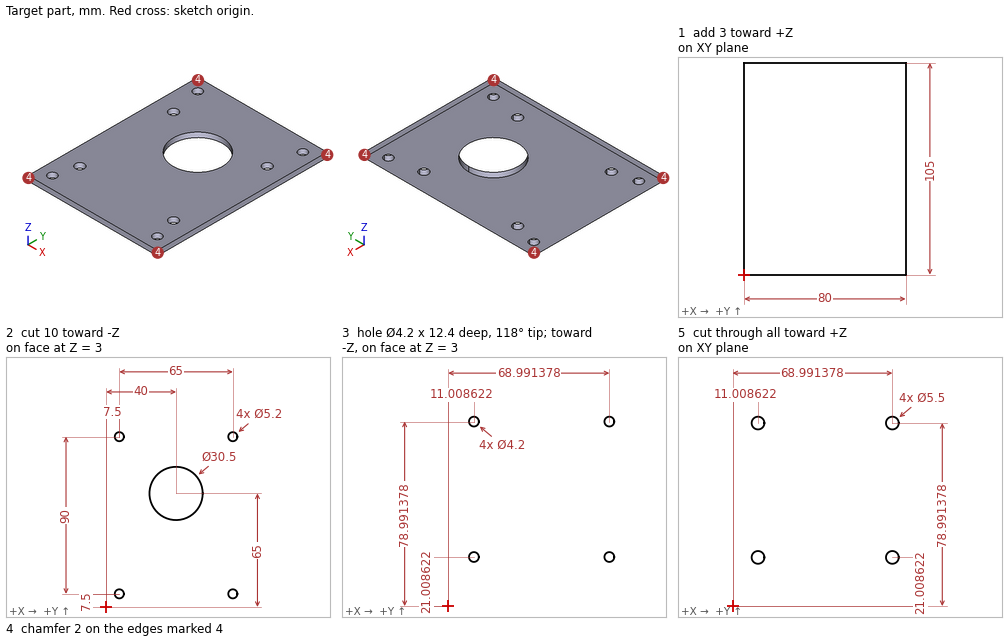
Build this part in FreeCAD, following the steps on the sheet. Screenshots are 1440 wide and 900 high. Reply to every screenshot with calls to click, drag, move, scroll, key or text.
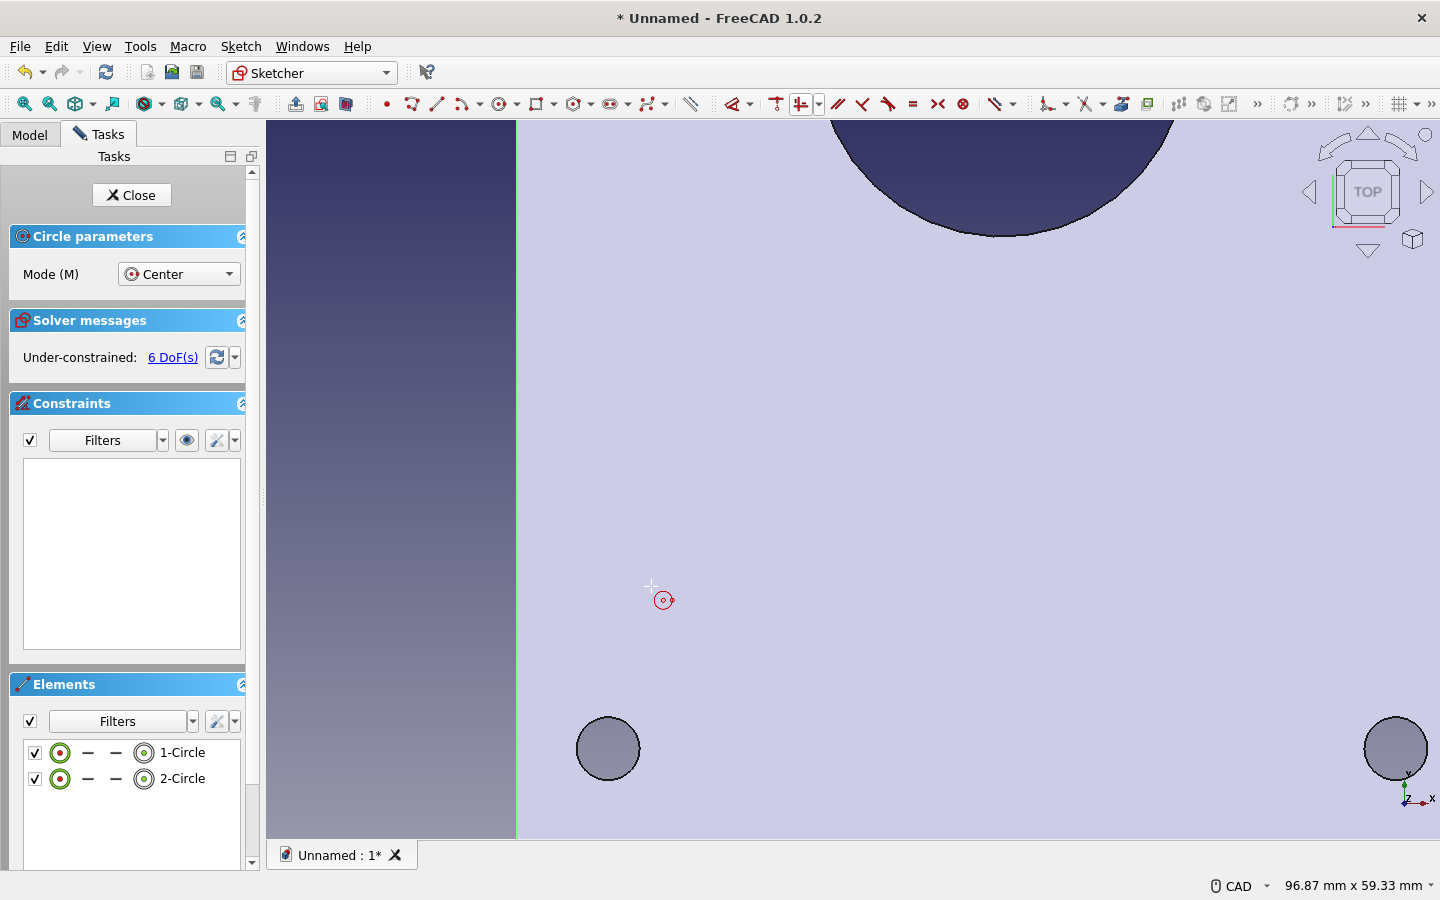
click(651, 585)
click(669, 567)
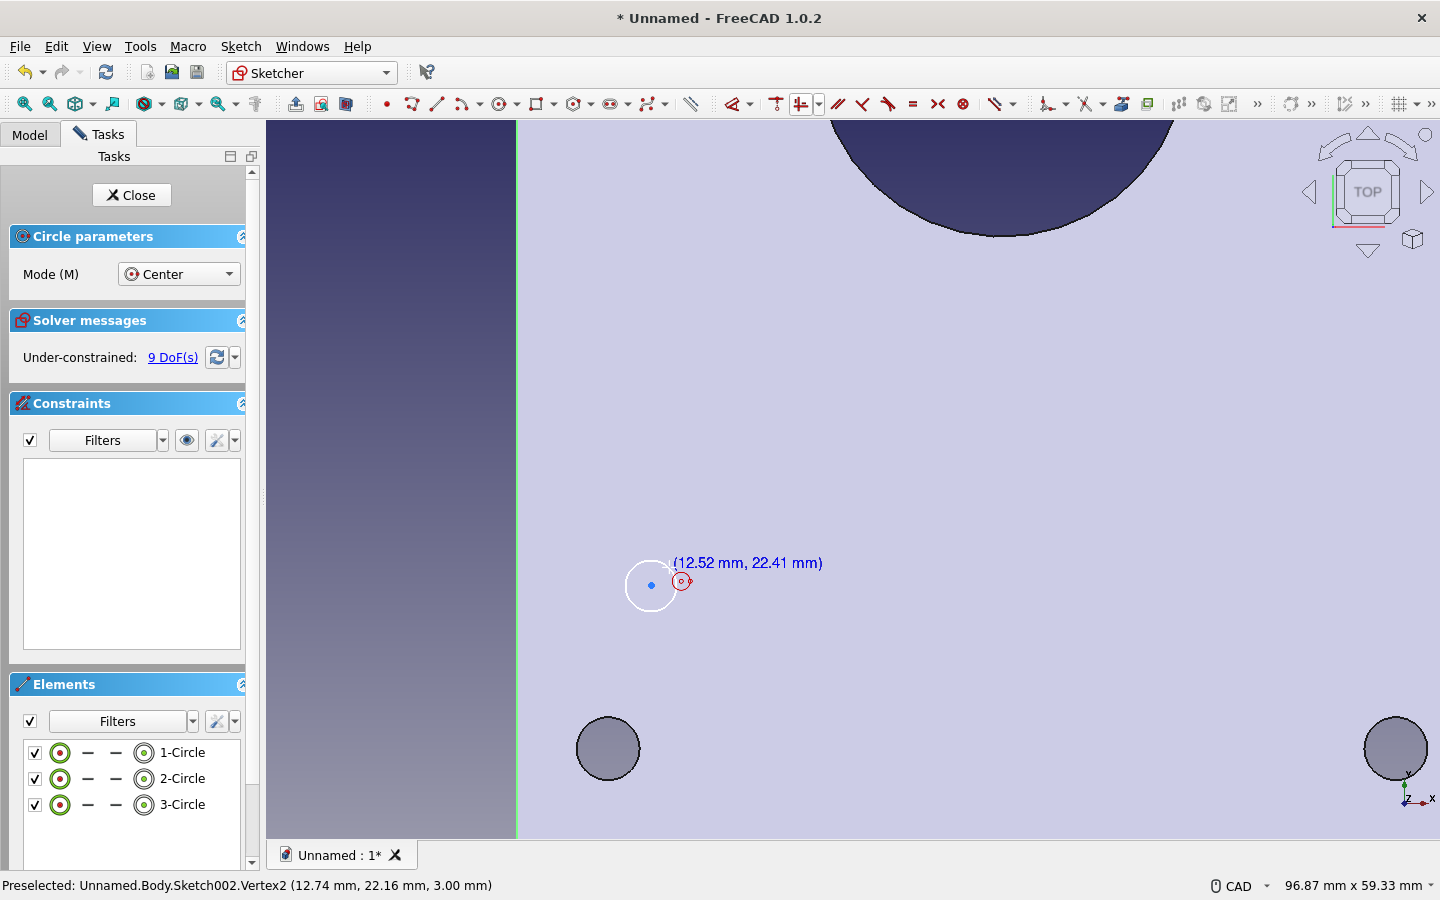
scroll(651, 587, down, 4)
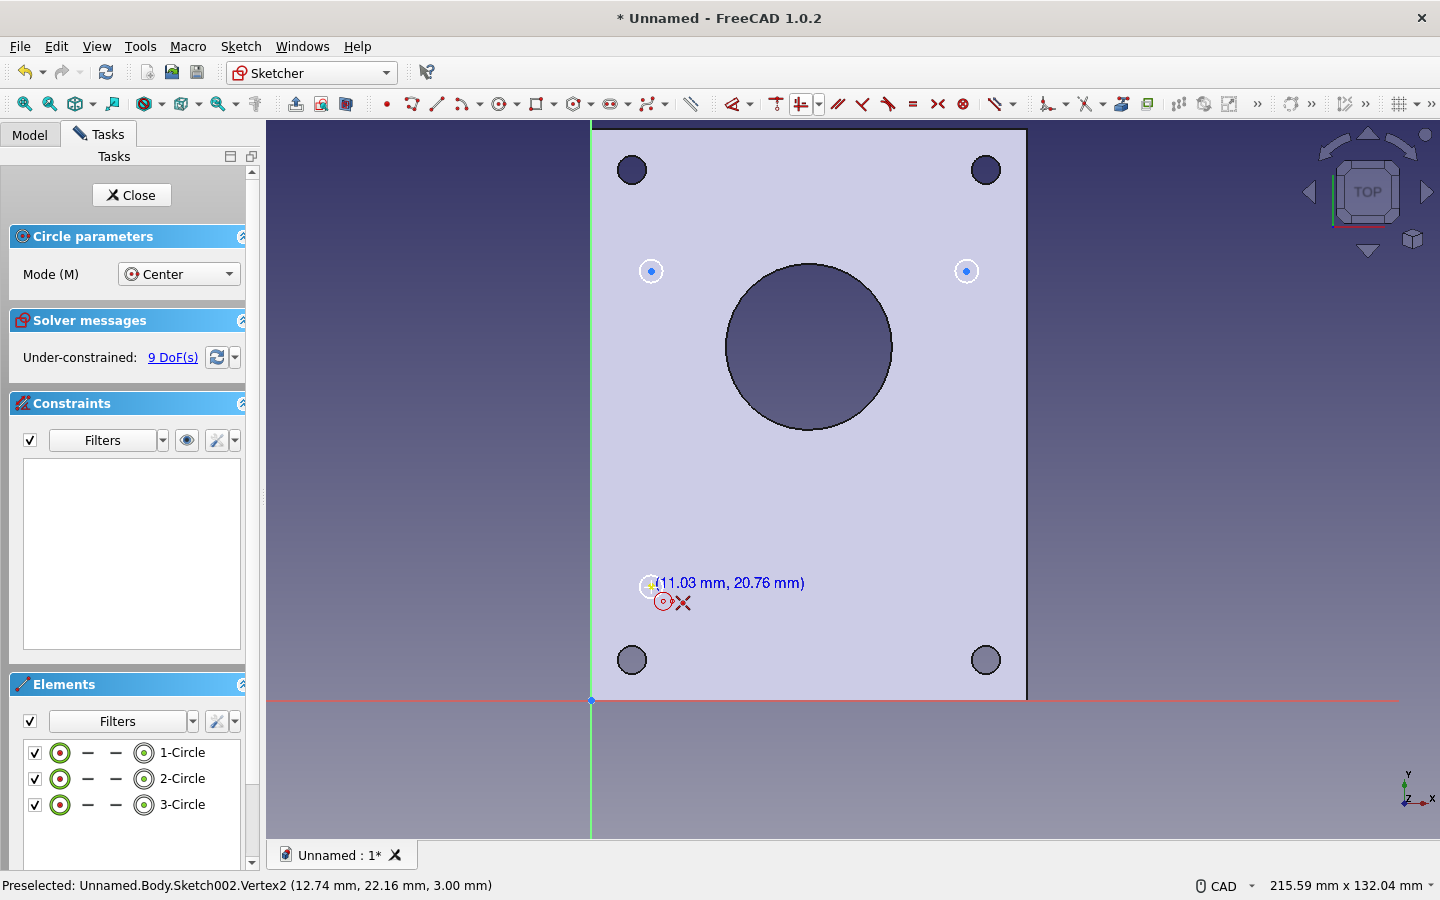
scroll(967, 586, up, 4)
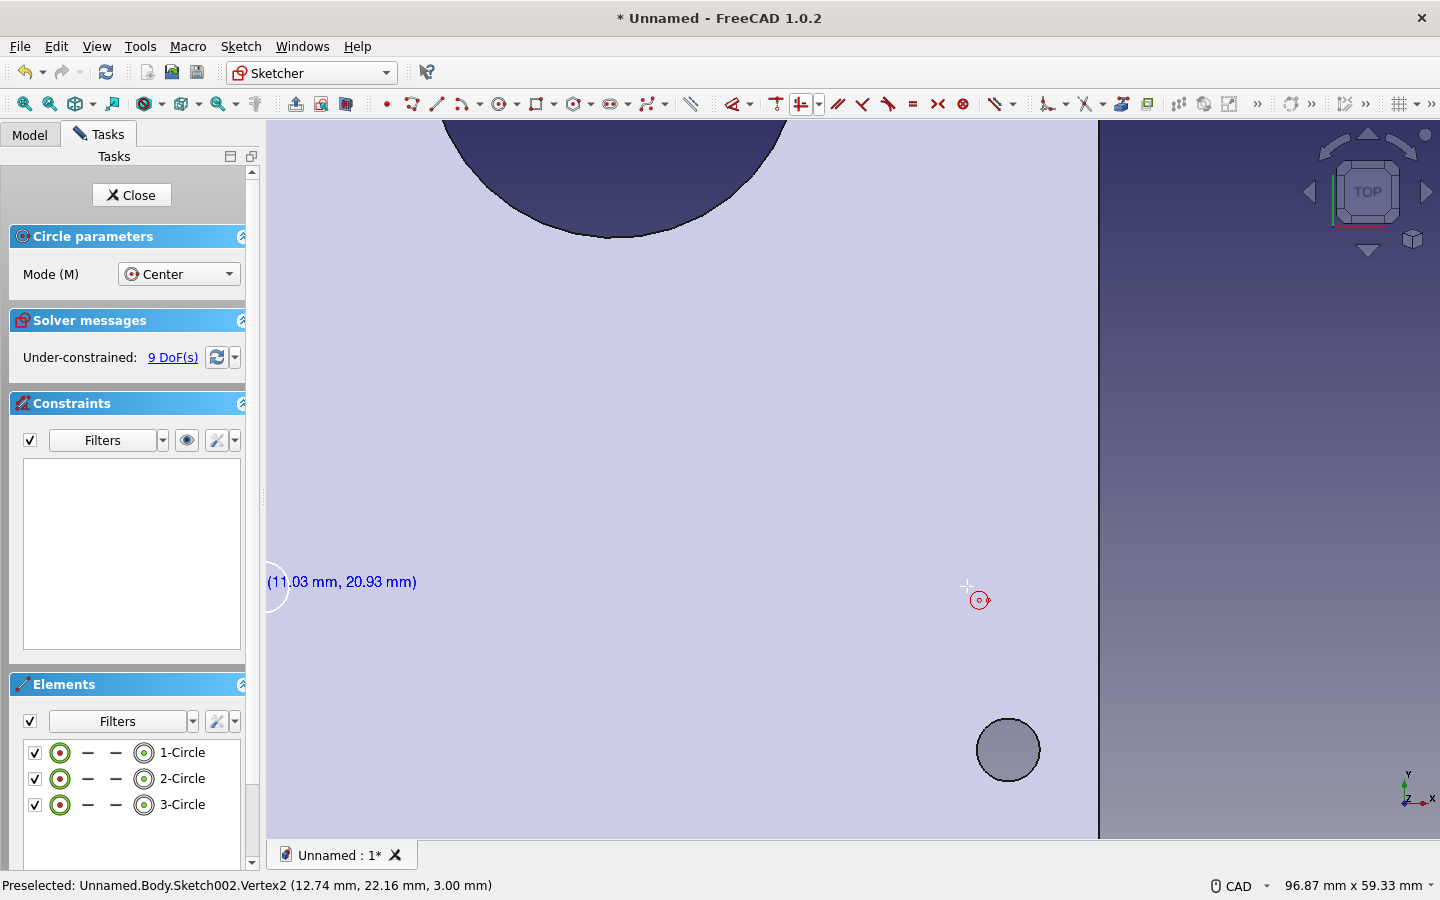
click(966, 586)
click(984, 568)
key(Escape)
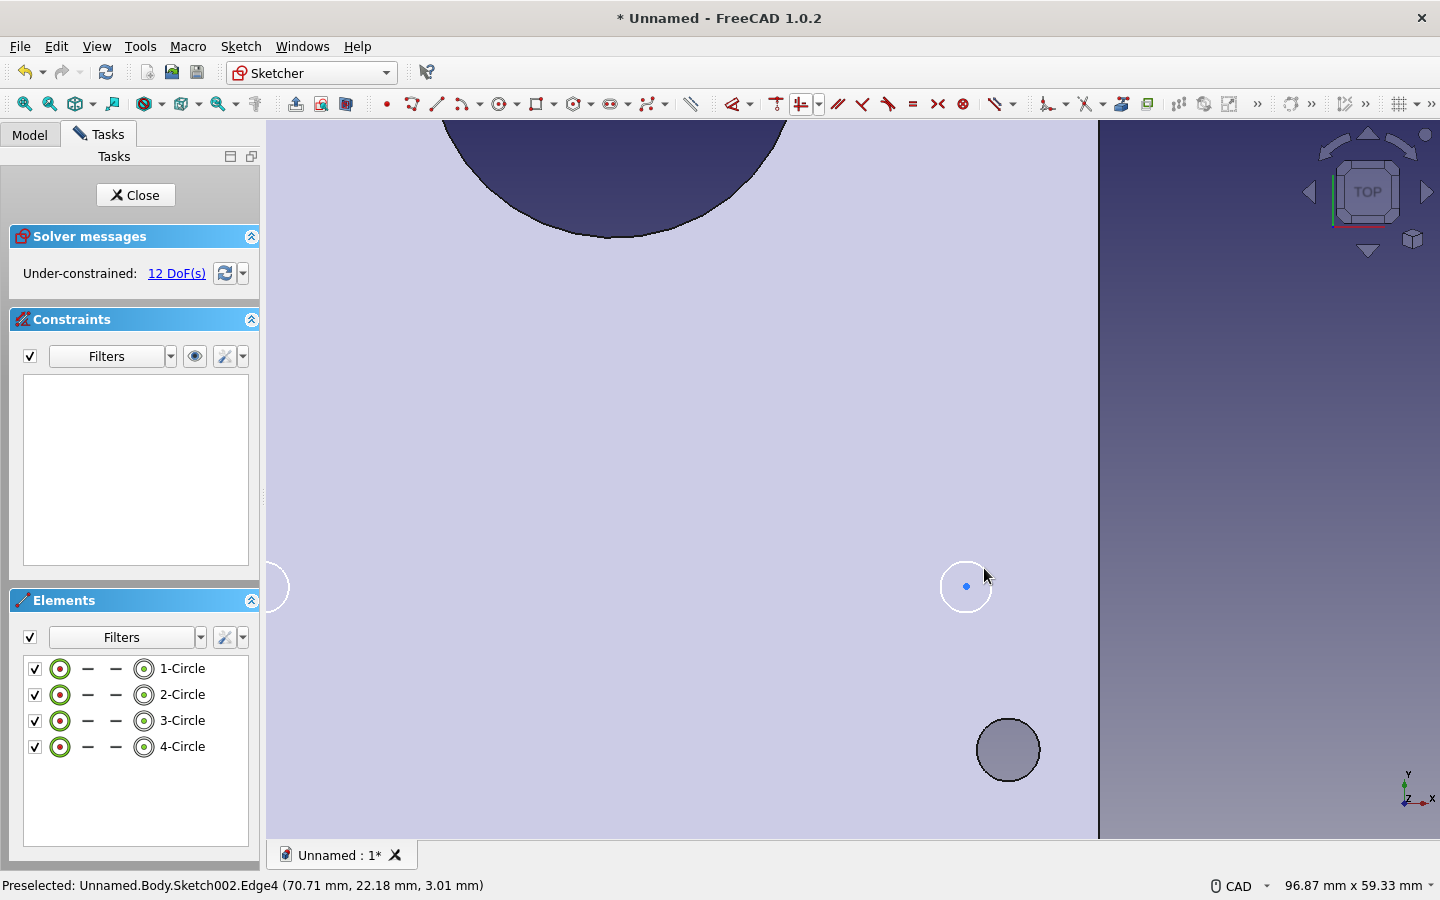
scroll(967, 586, down, 4)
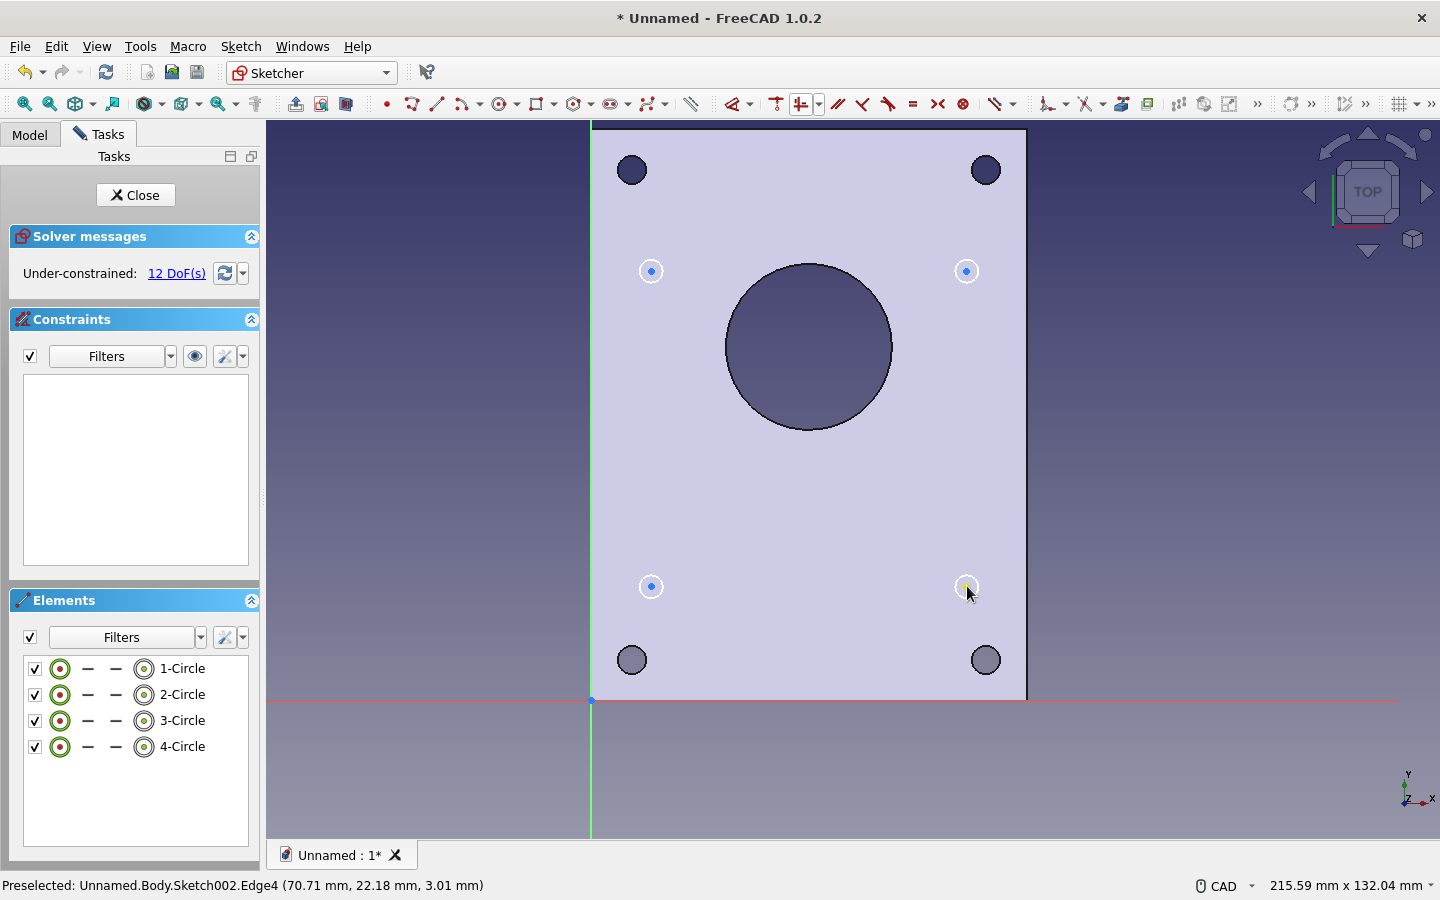
click(659, 263)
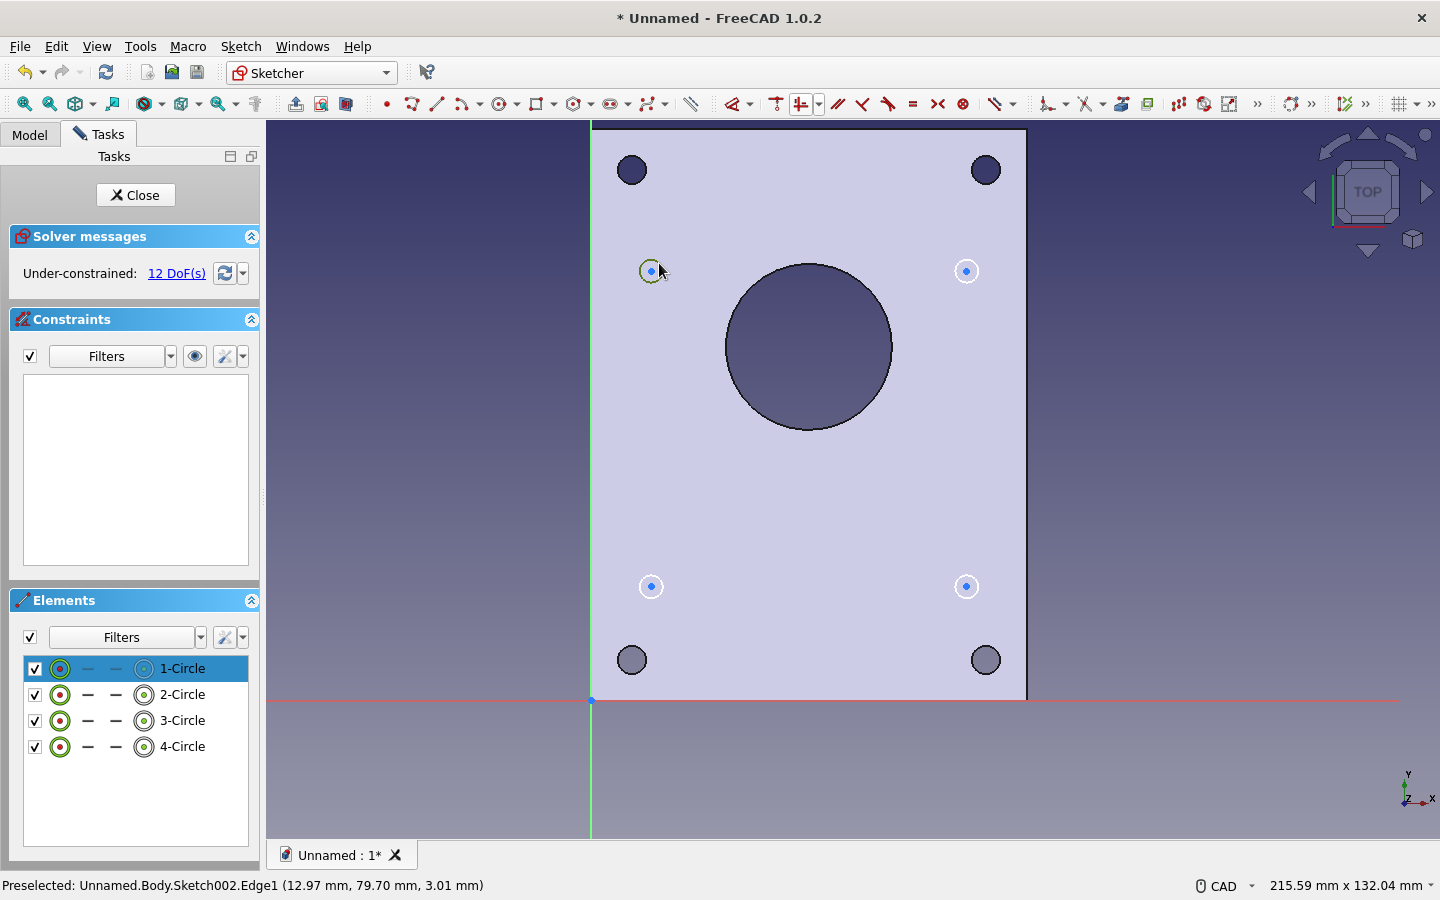
click(975, 263)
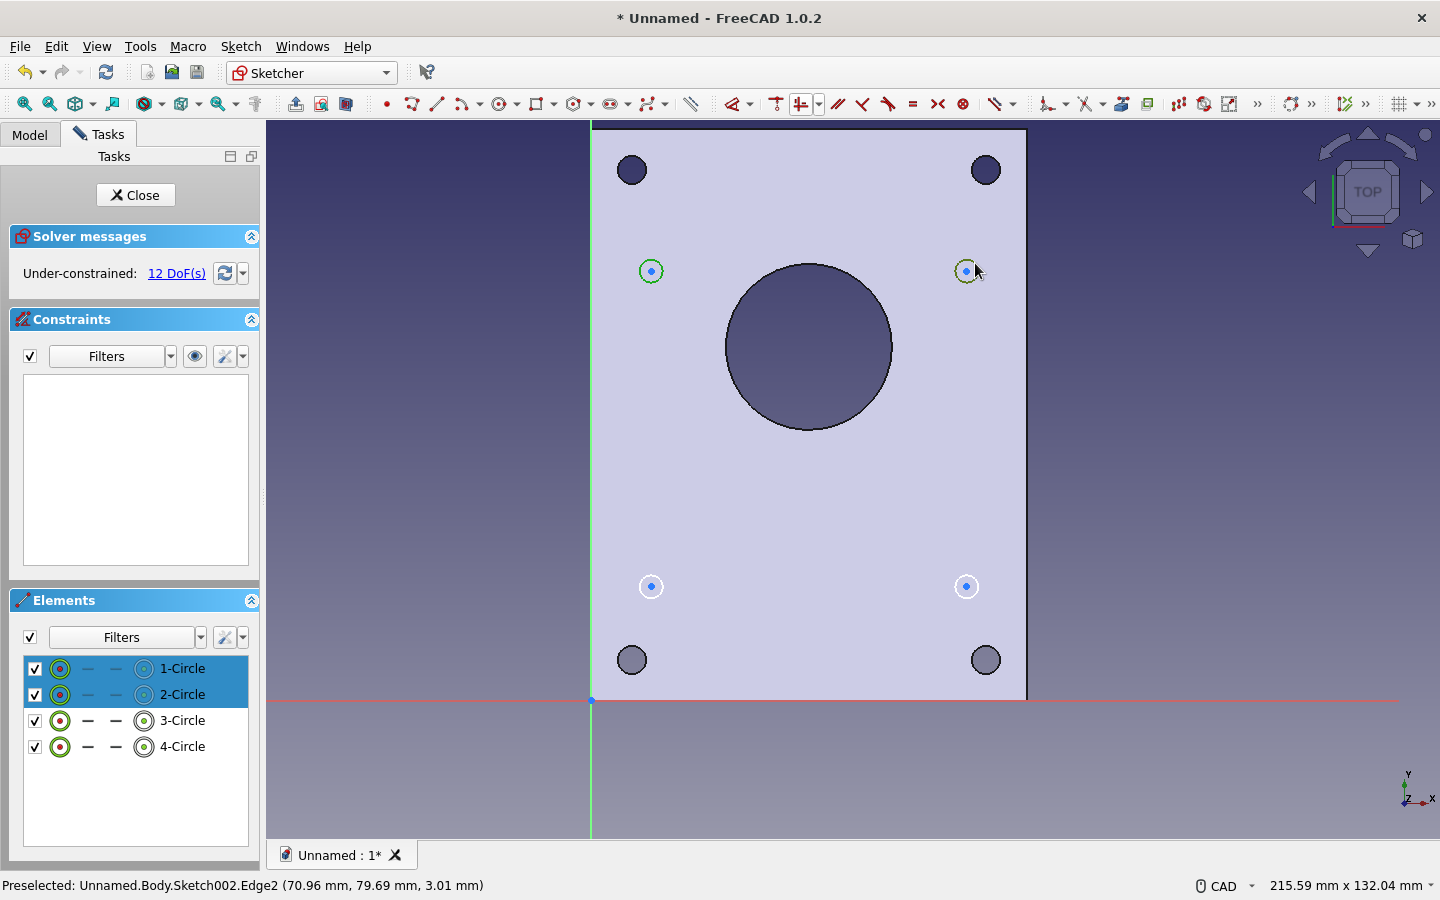
click(659, 579)